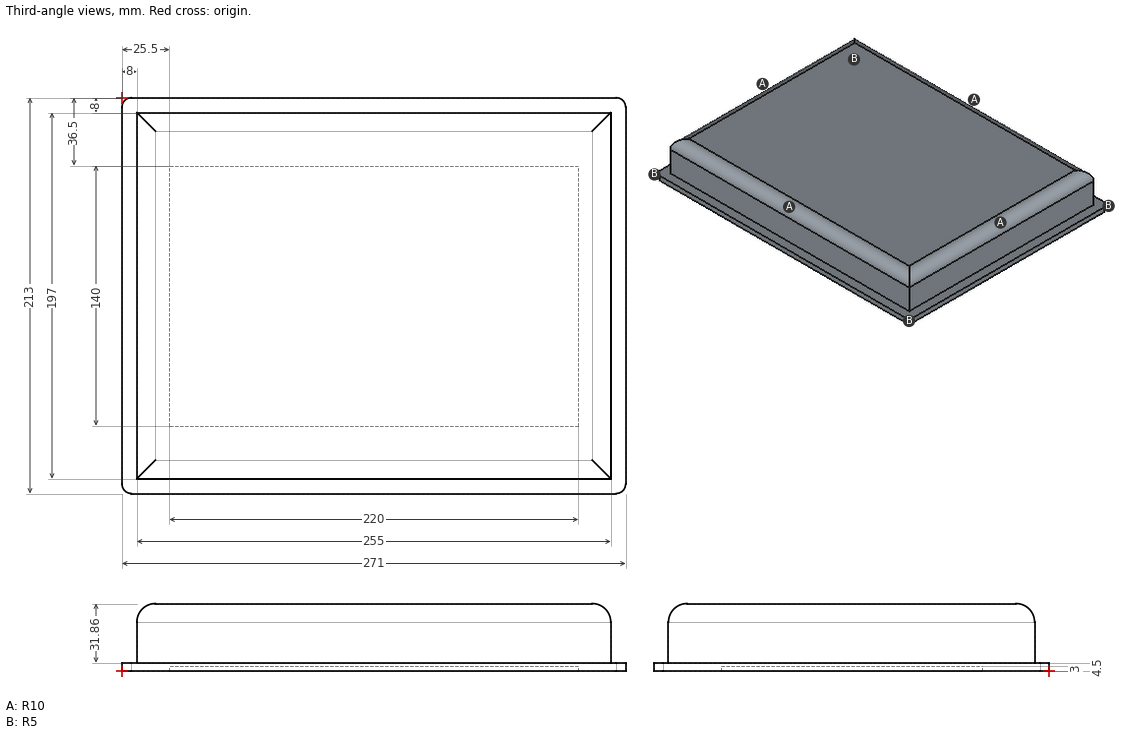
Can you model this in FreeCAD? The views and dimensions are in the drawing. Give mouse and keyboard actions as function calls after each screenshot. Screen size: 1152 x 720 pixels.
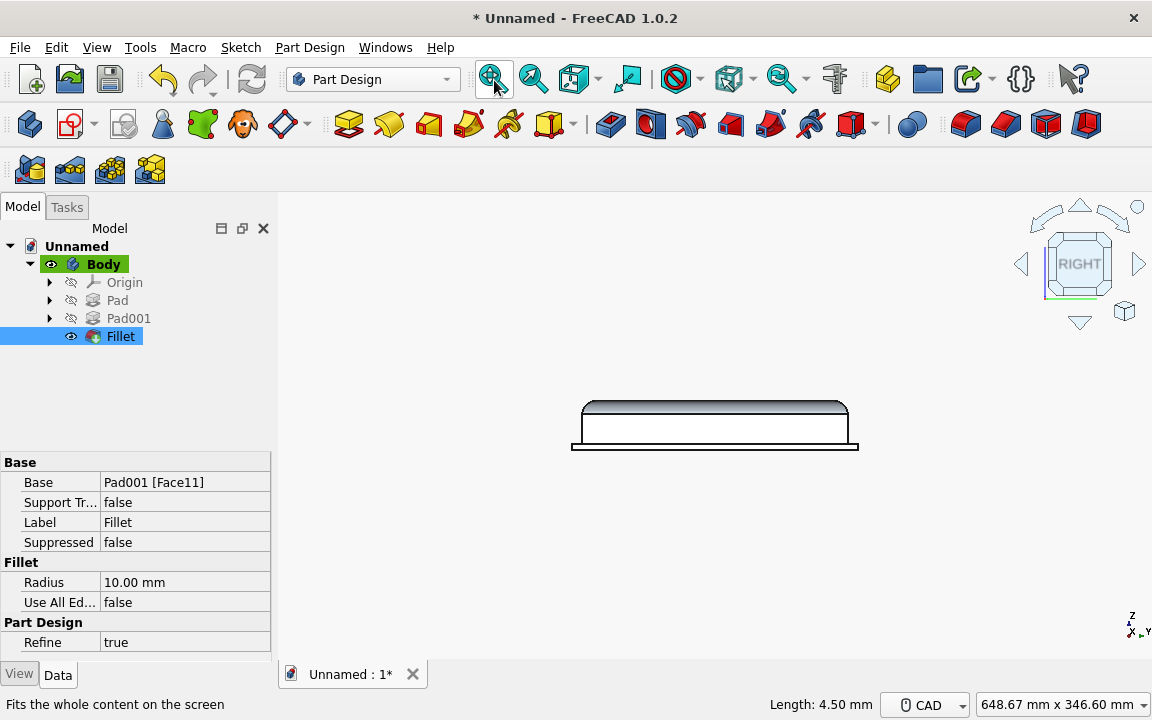
scroll(858, 446, up, 10)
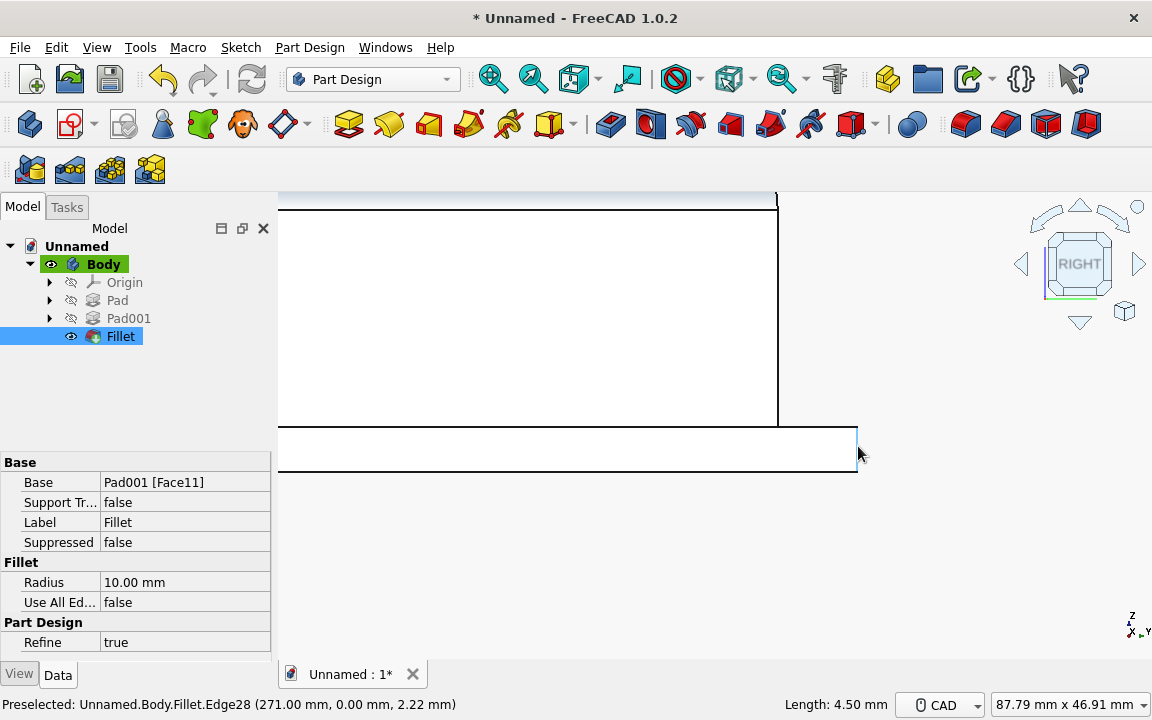
click(857, 449, ctrl)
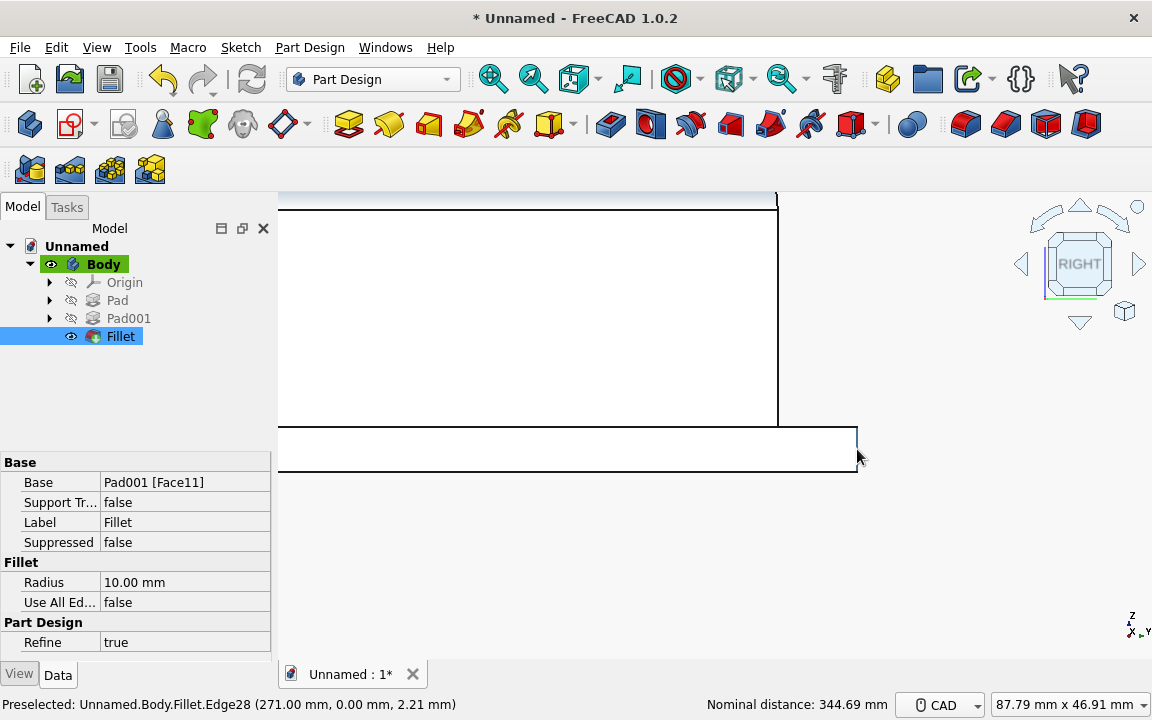
click(494, 80)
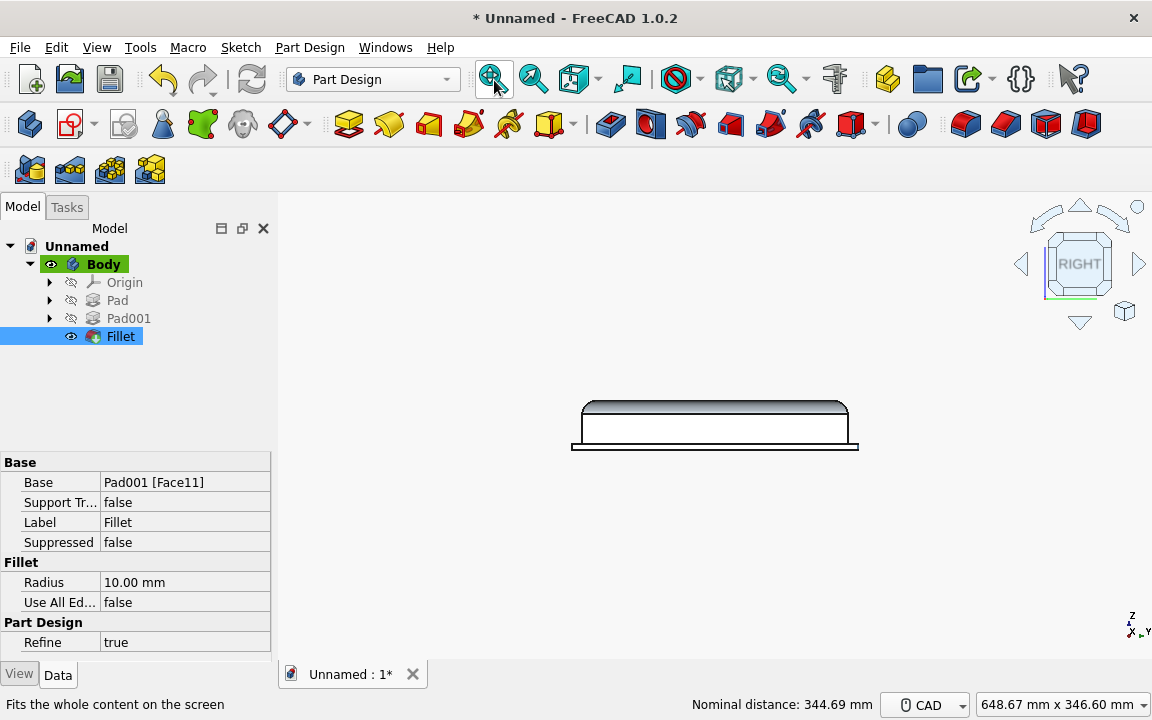
key(5)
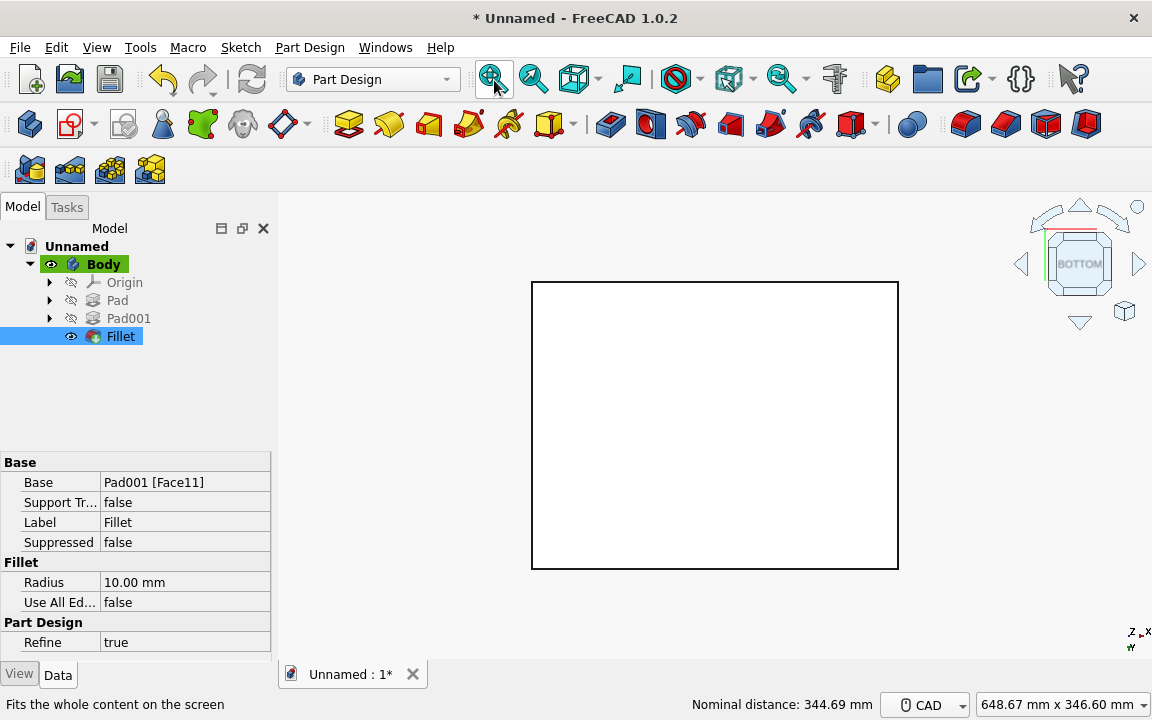
scroll(532, 568, up, 10)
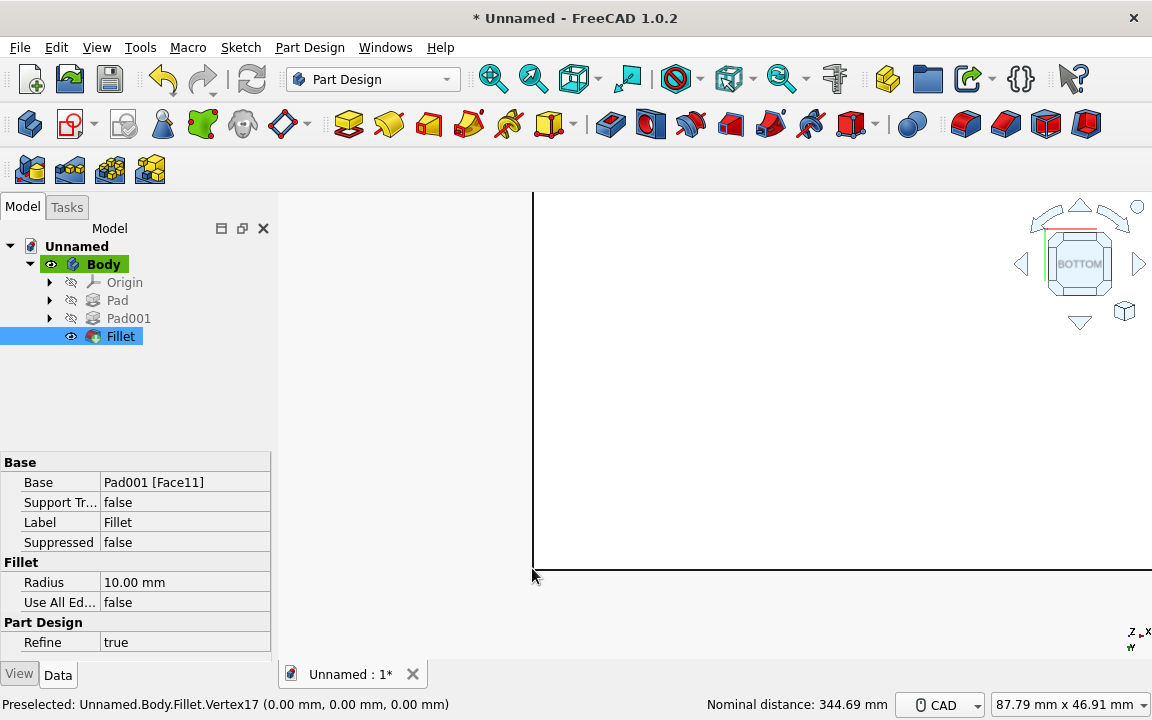
click(494, 80)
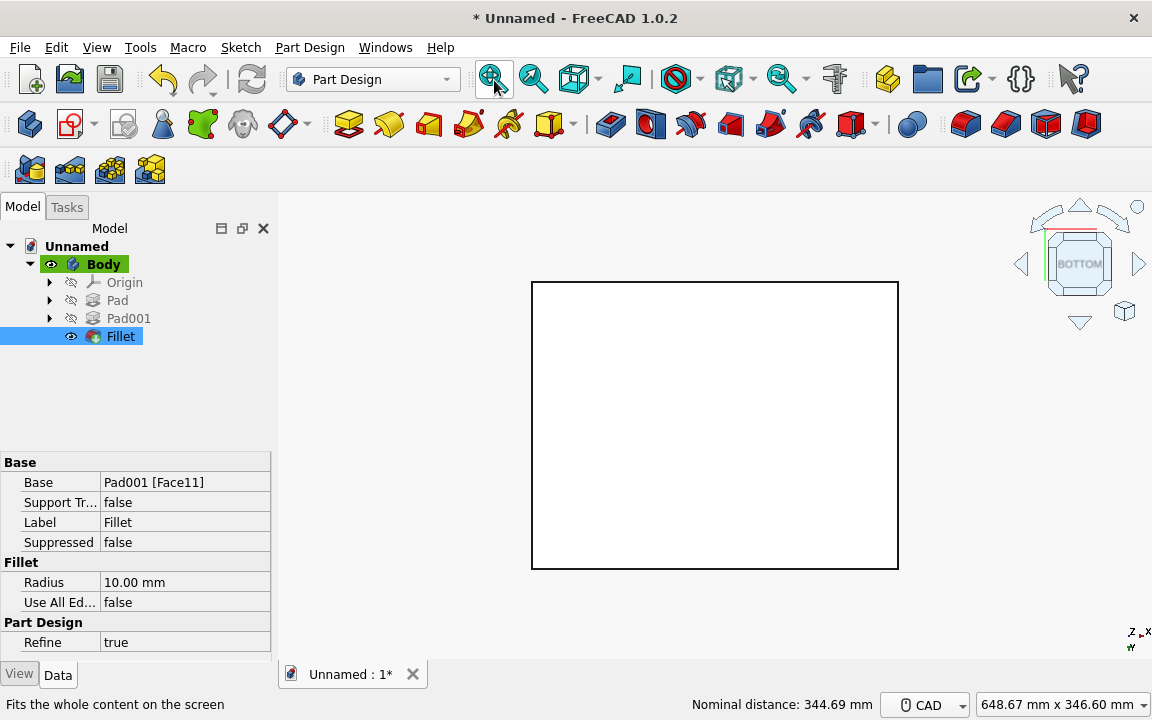
key(4)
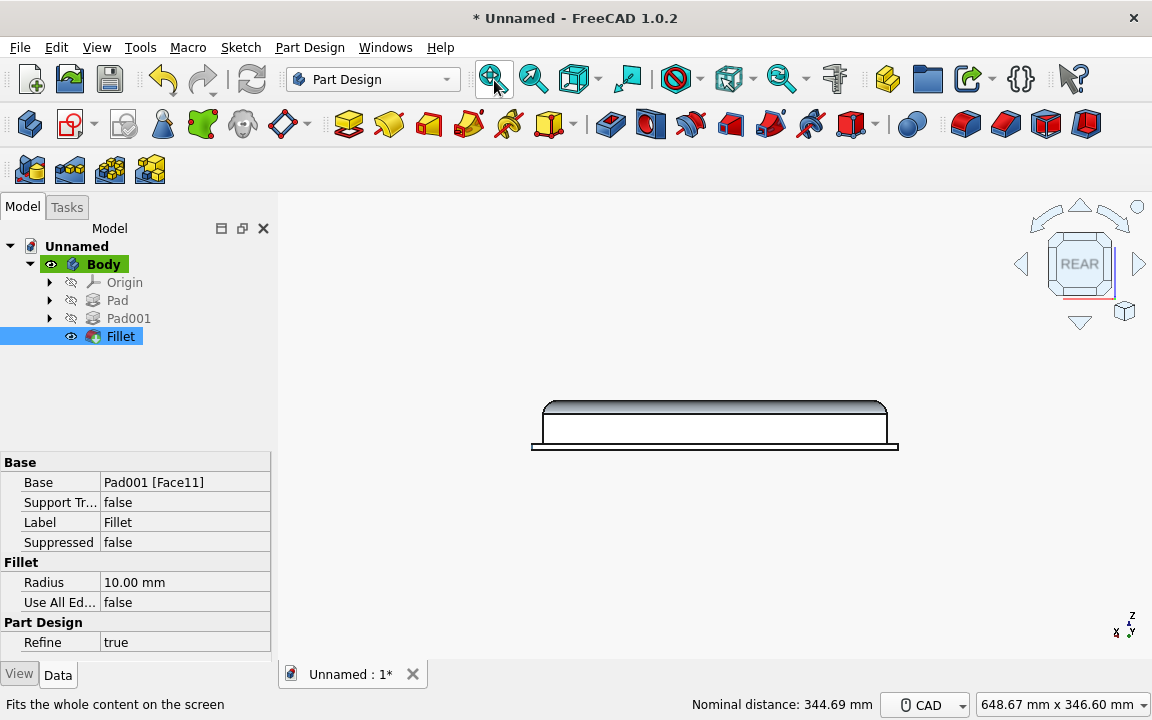
click(494, 80)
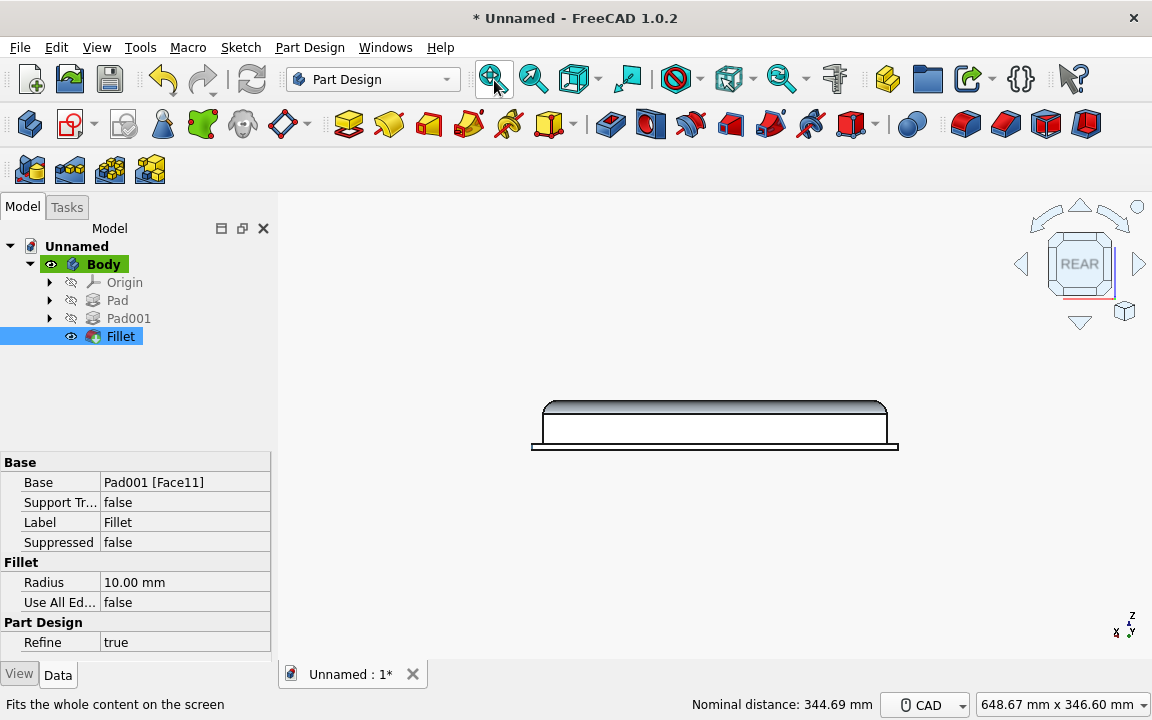
scroll(898, 446, up, 10)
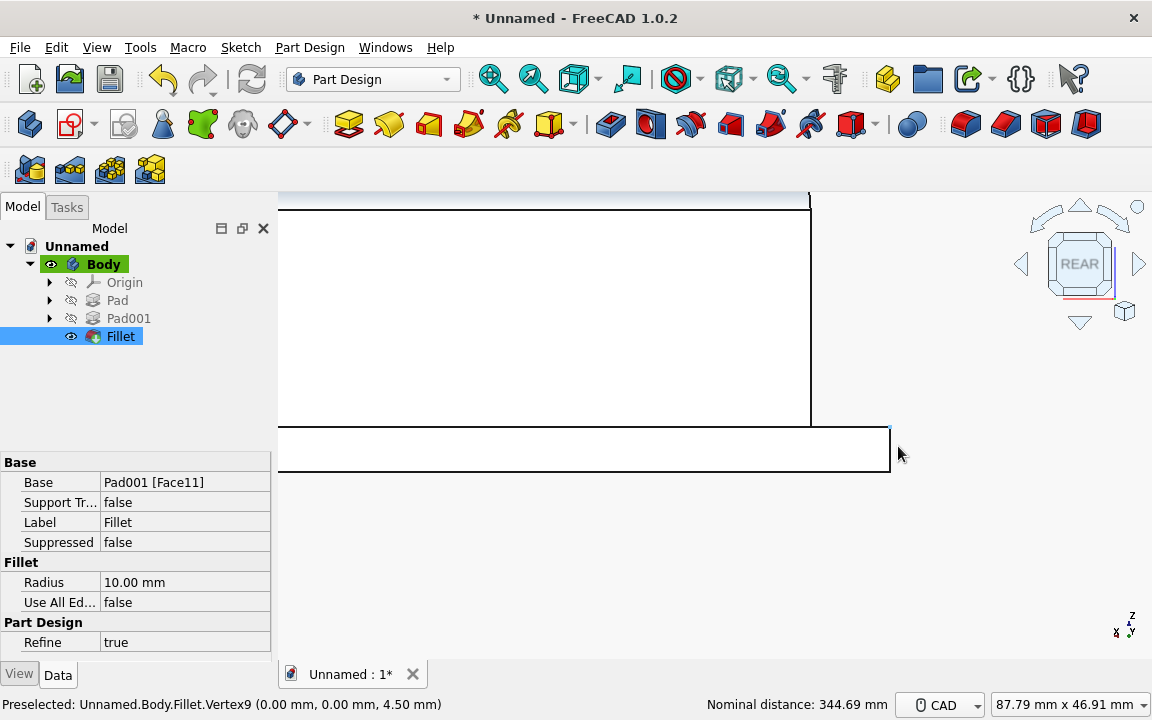
click(494, 80)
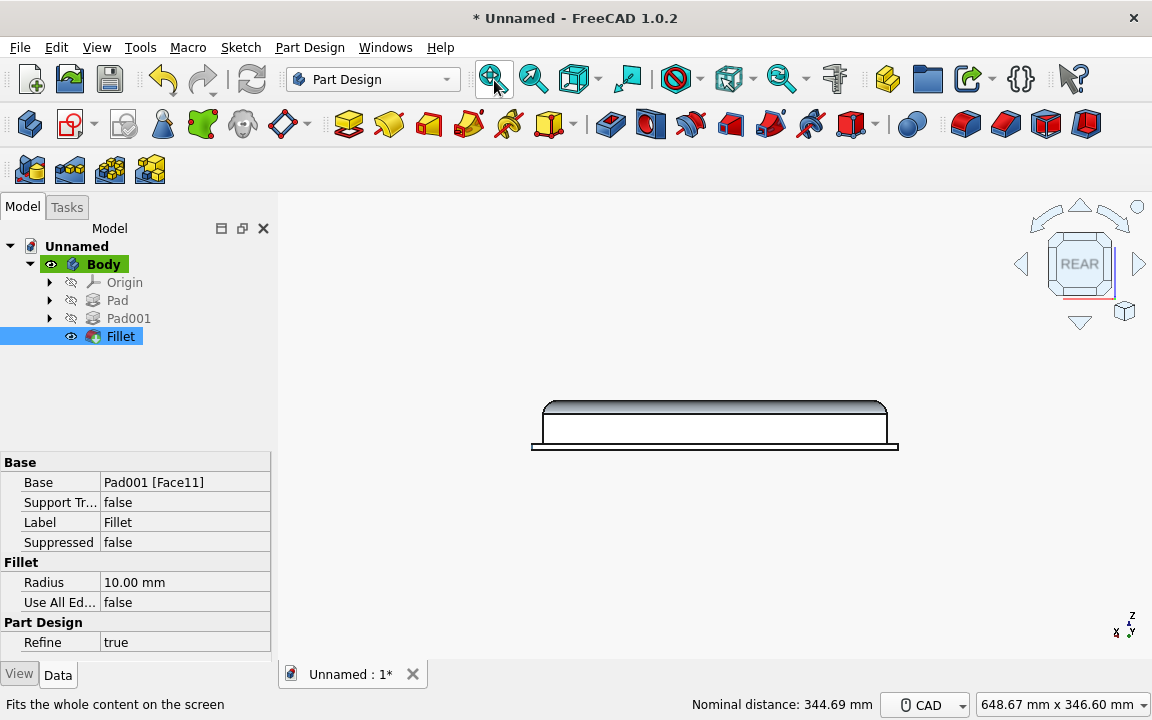
key(6)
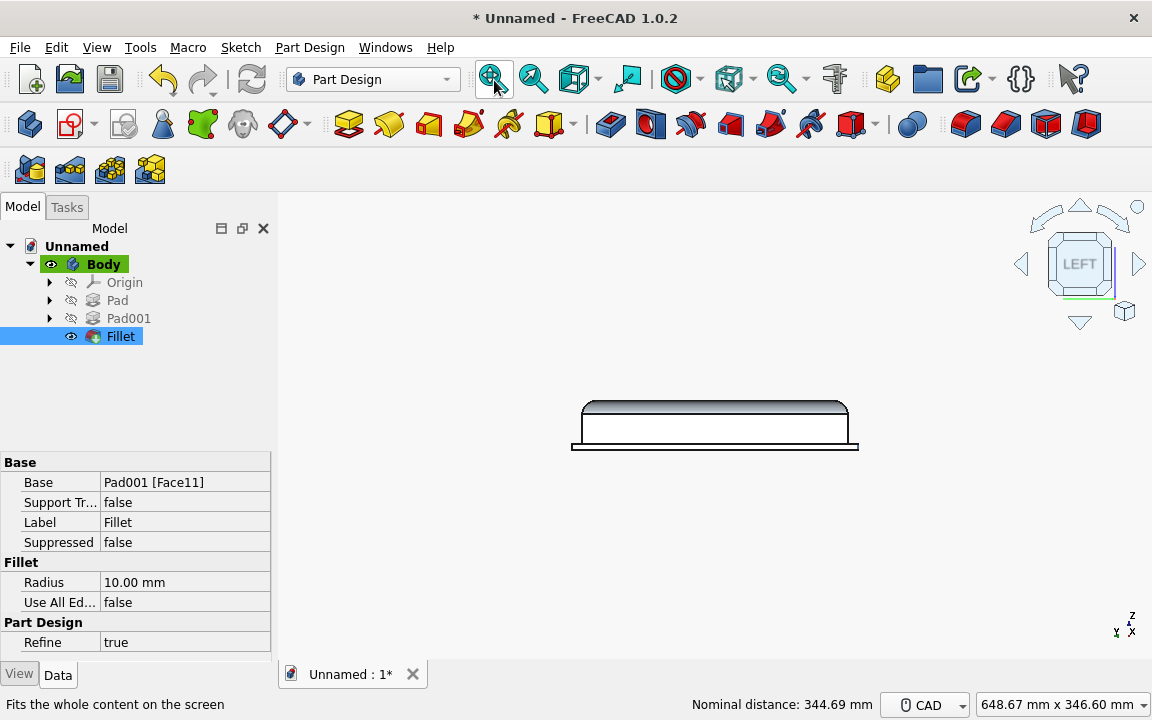
click(494, 80)